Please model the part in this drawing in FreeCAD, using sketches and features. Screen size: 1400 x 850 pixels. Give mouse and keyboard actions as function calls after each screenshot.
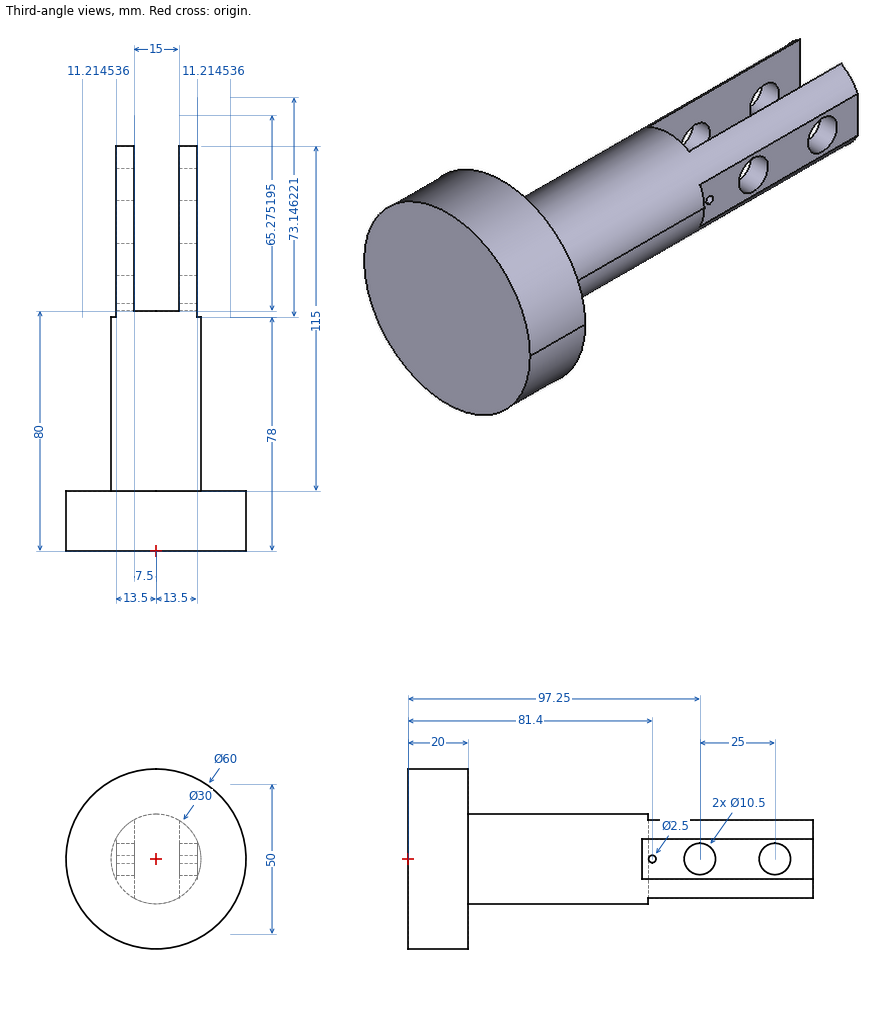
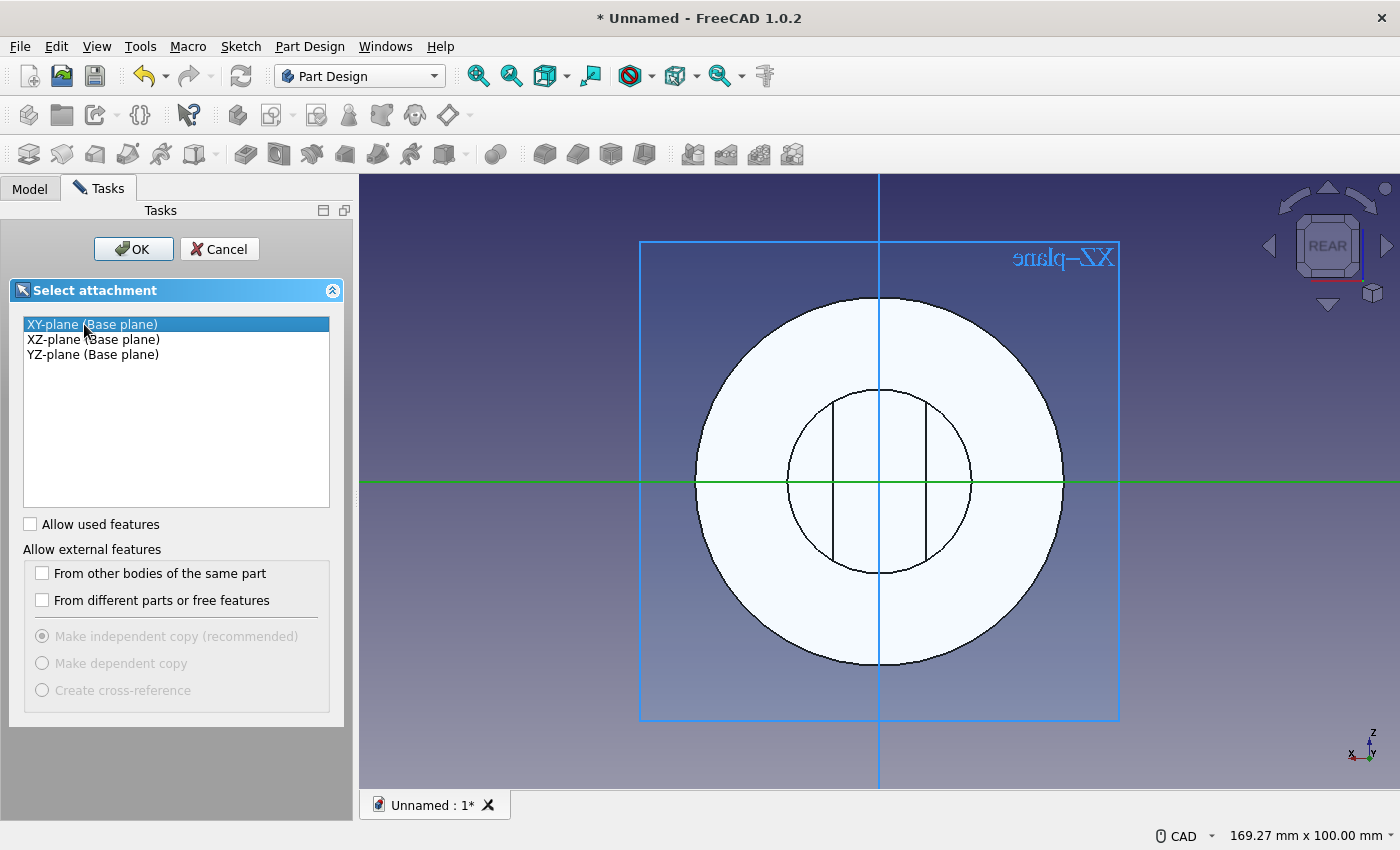
click(134, 249)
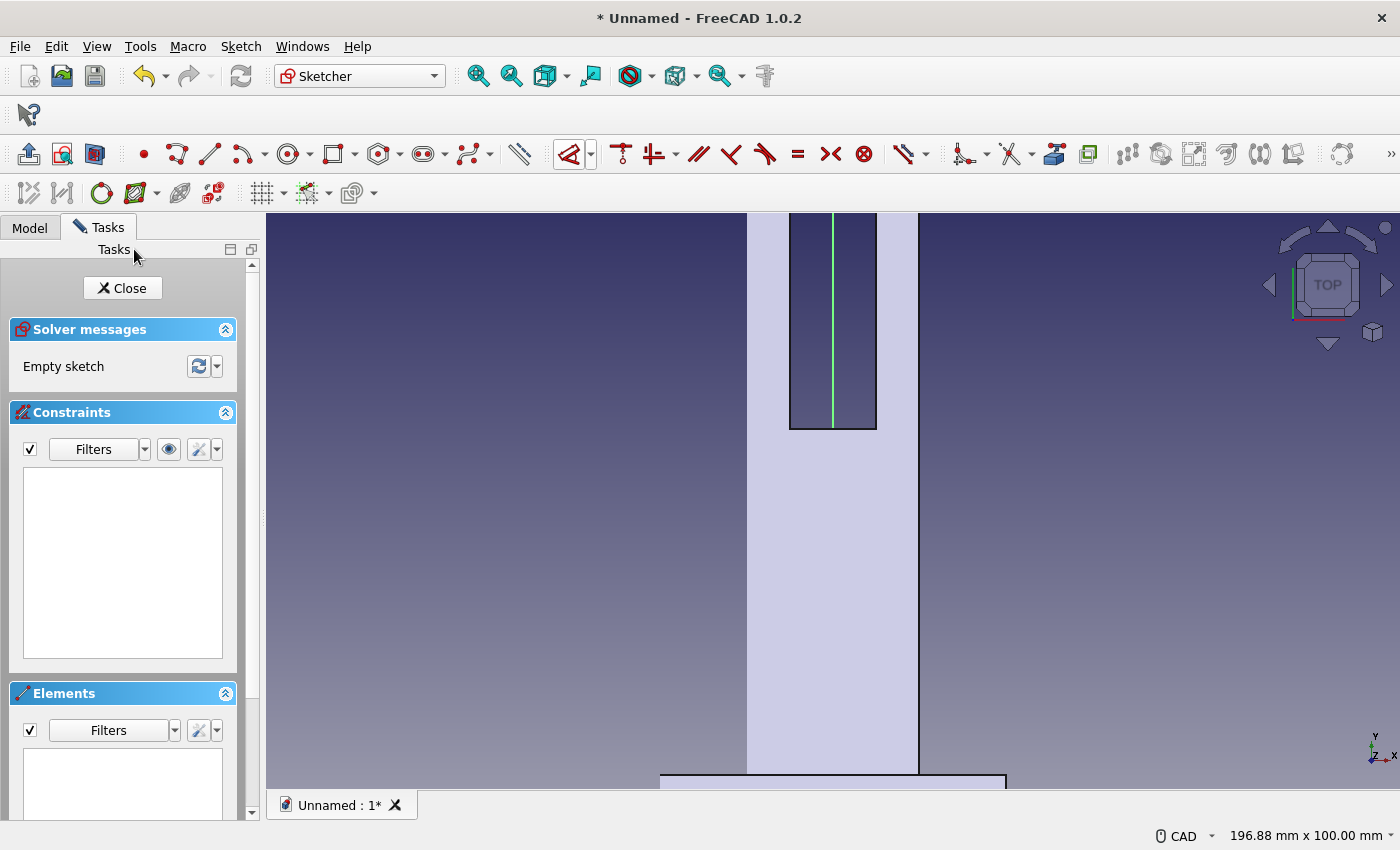
click(95, 154)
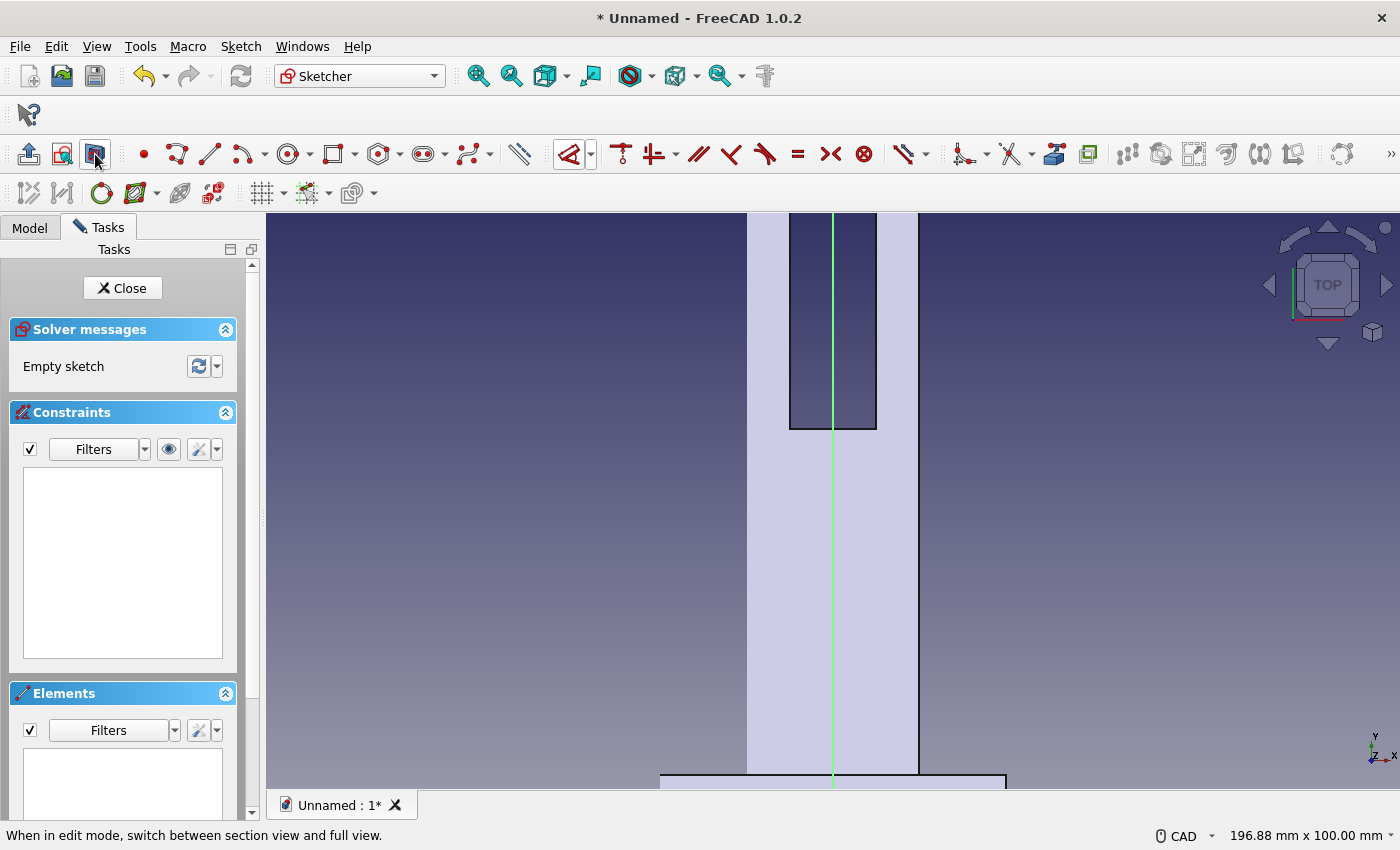
scroll(709, 539, down, 4)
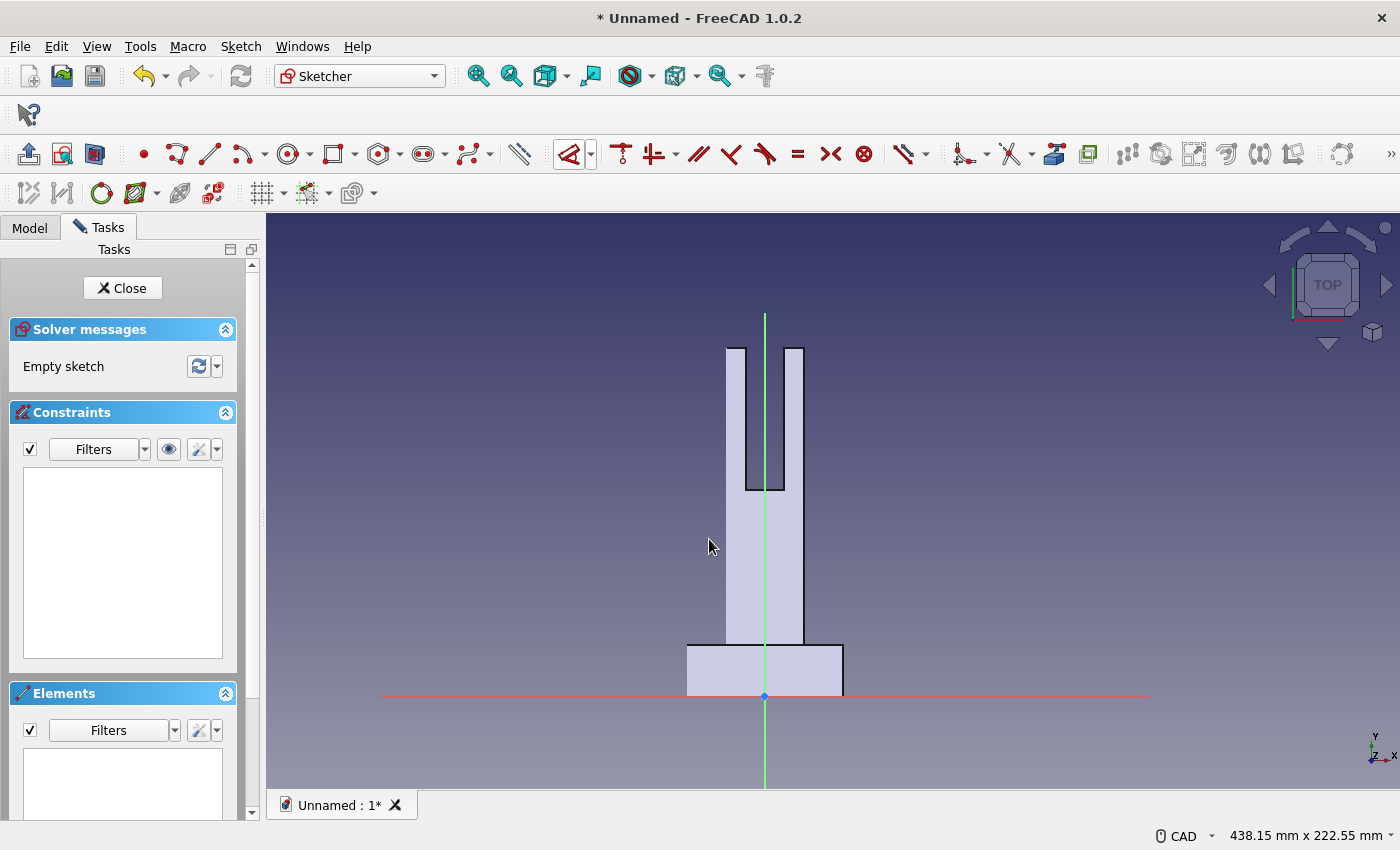
click(332, 154)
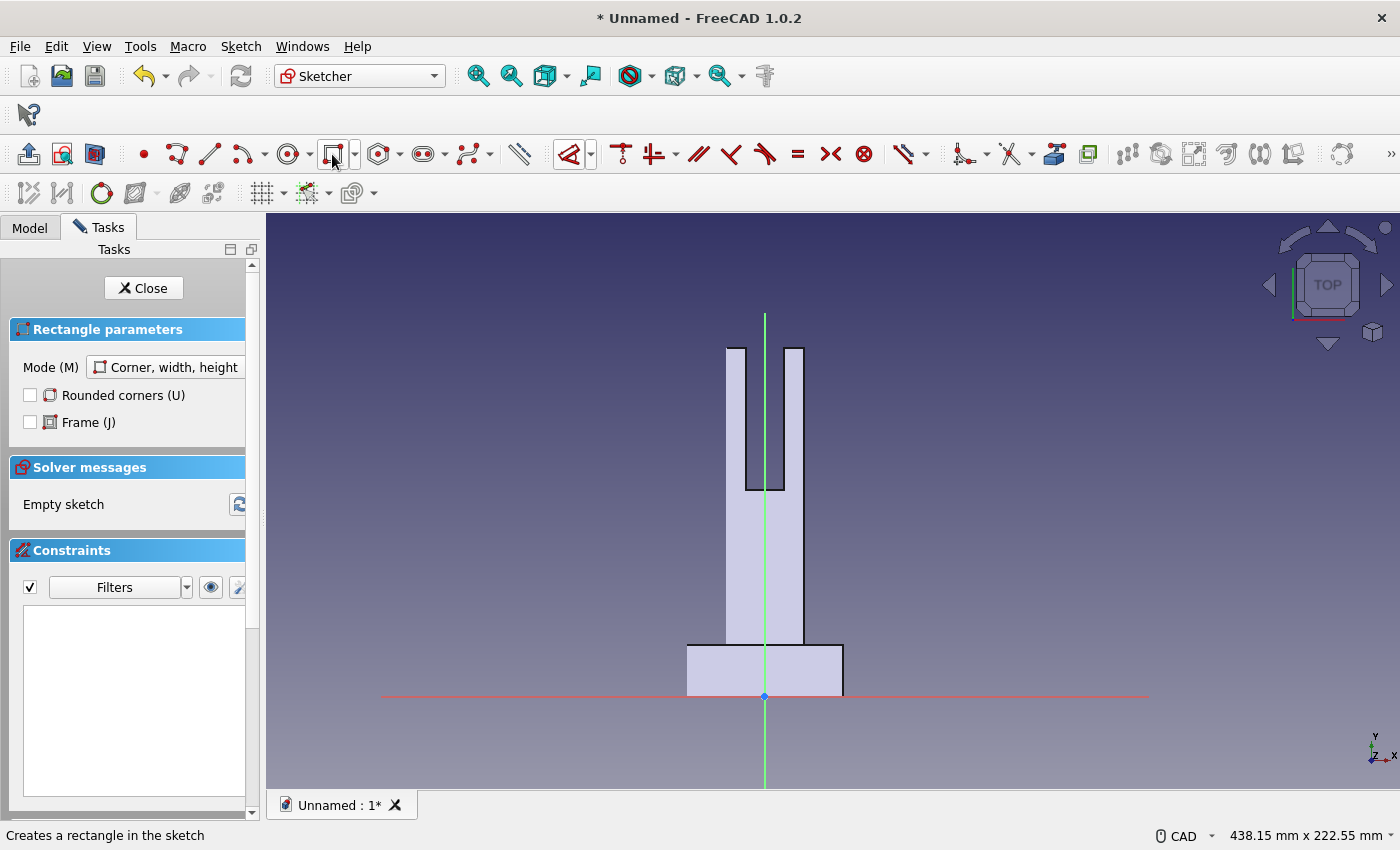
click(800, 306)
move(829, 495)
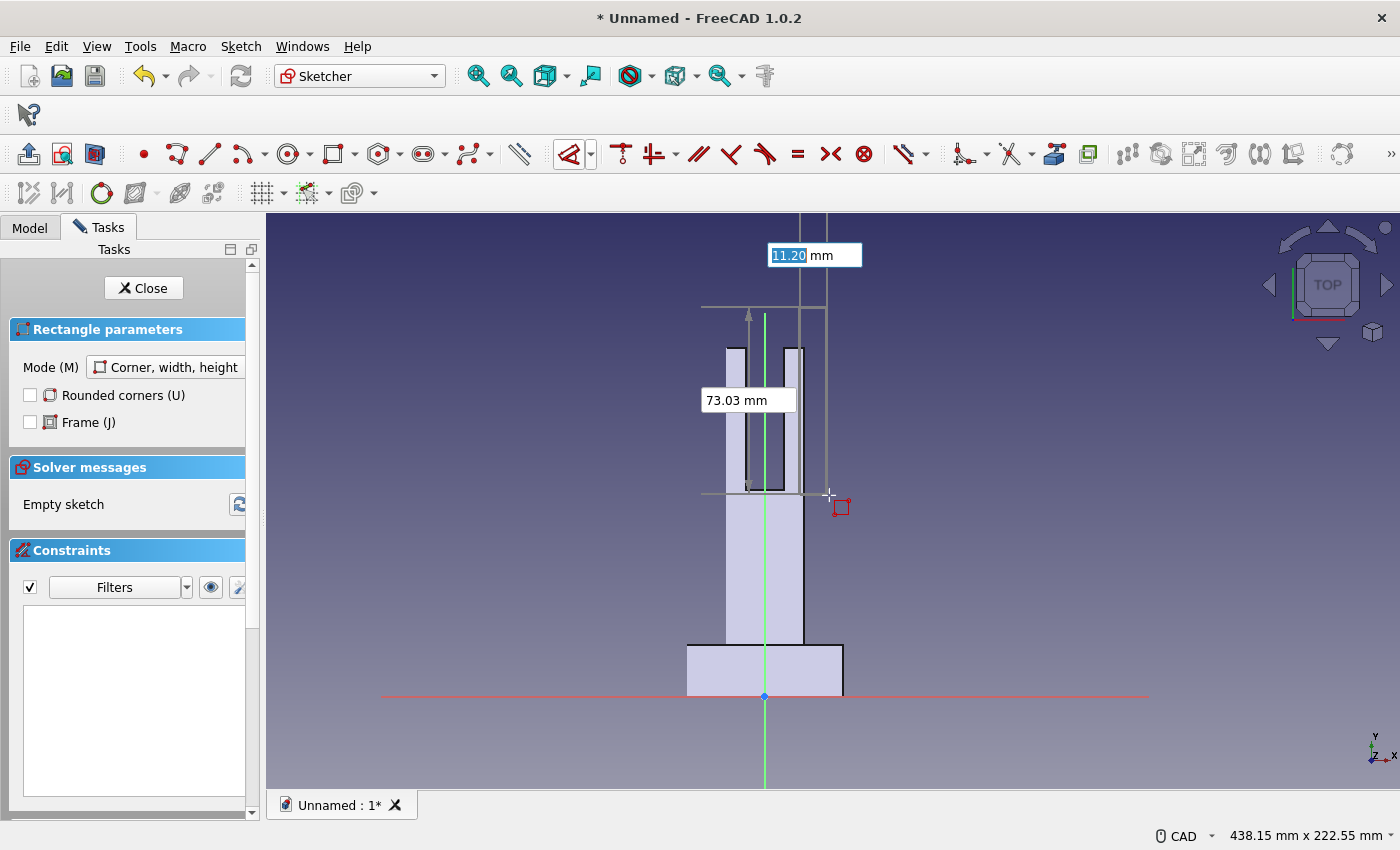
text(11.214536)
key(Tab)
text(73.146221)
key(Return)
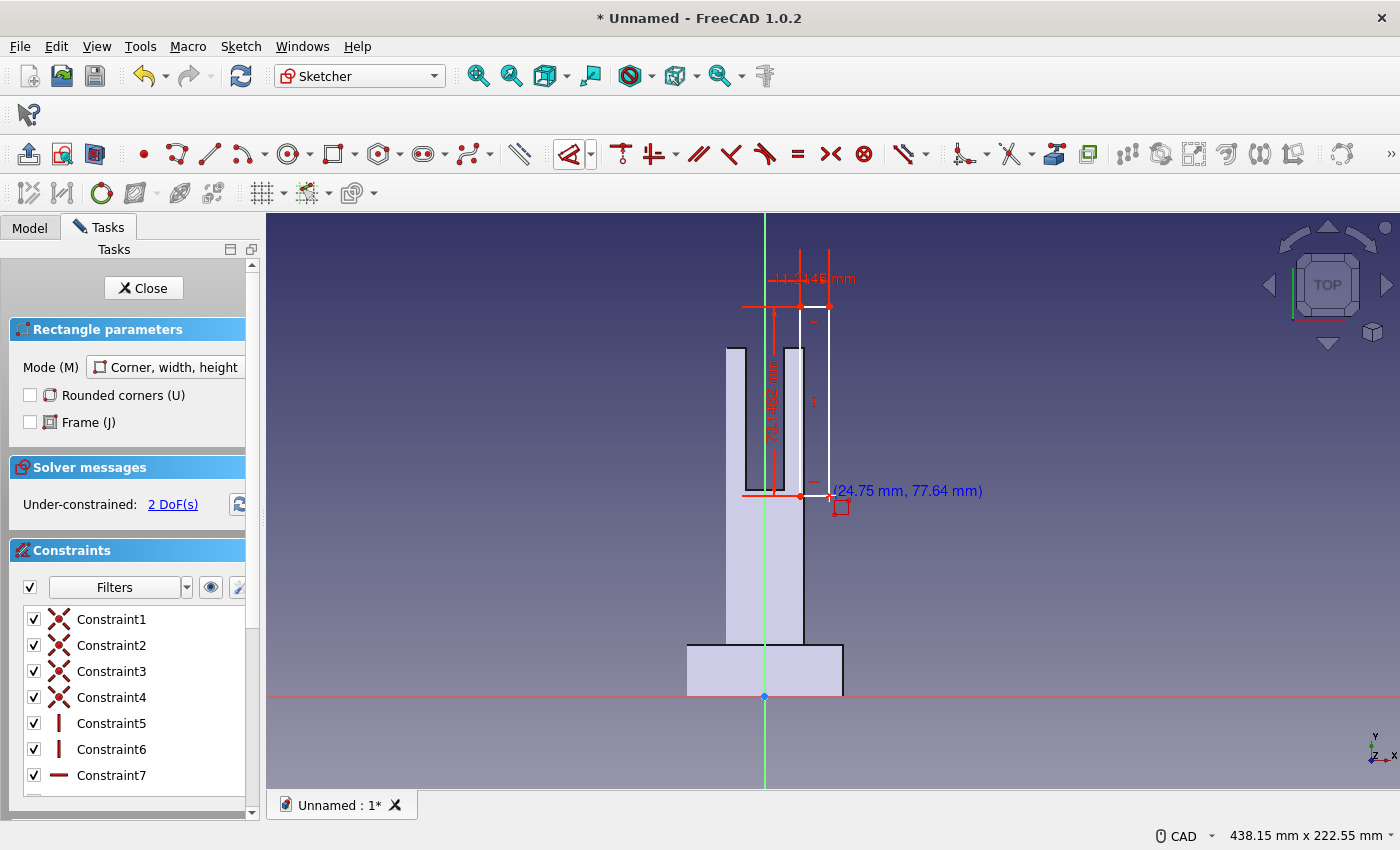
click(701, 306)
move(730, 495)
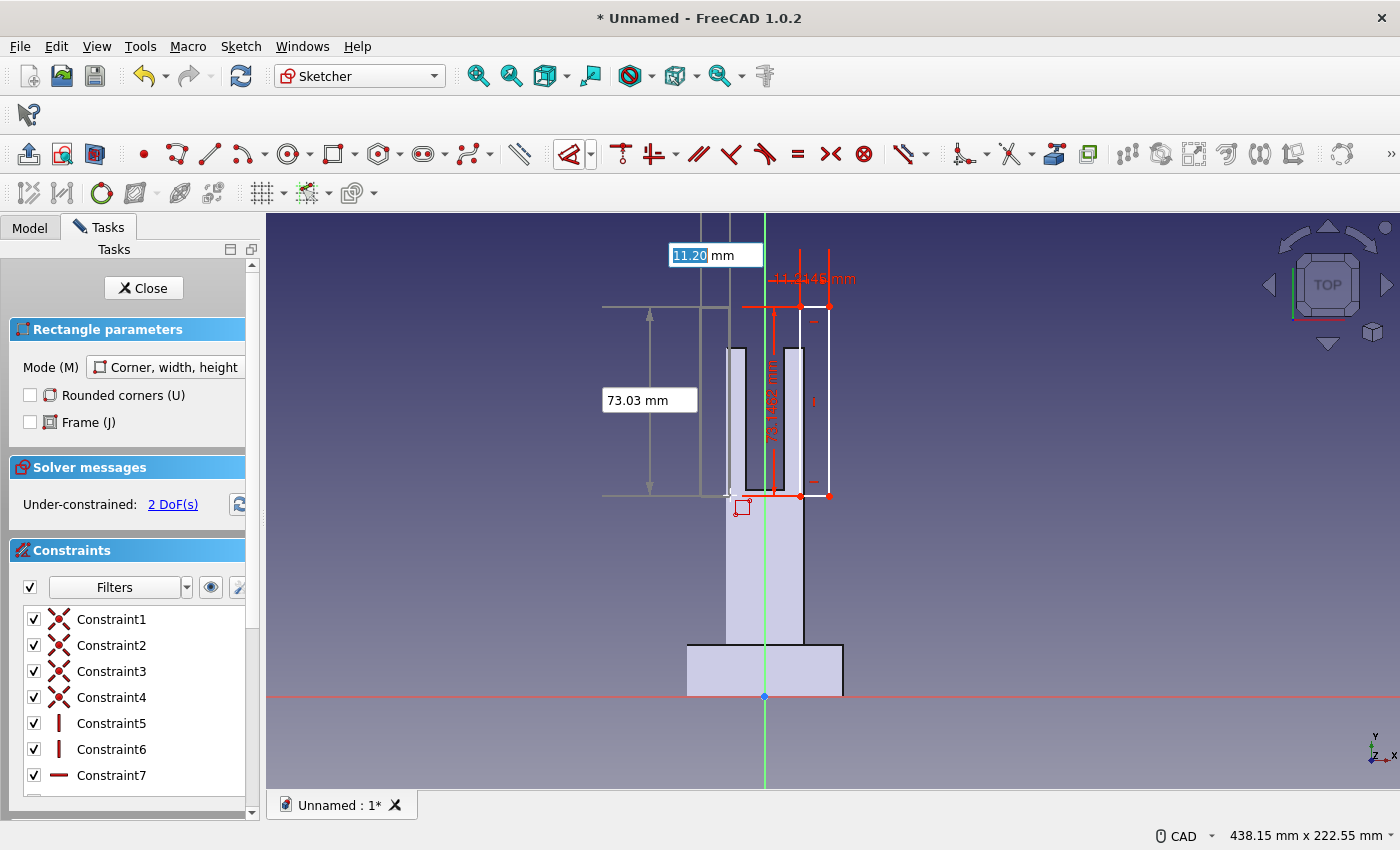
text(11.214536)
key(Tab)
text(73.146221)
key(Return)
key(Escape)